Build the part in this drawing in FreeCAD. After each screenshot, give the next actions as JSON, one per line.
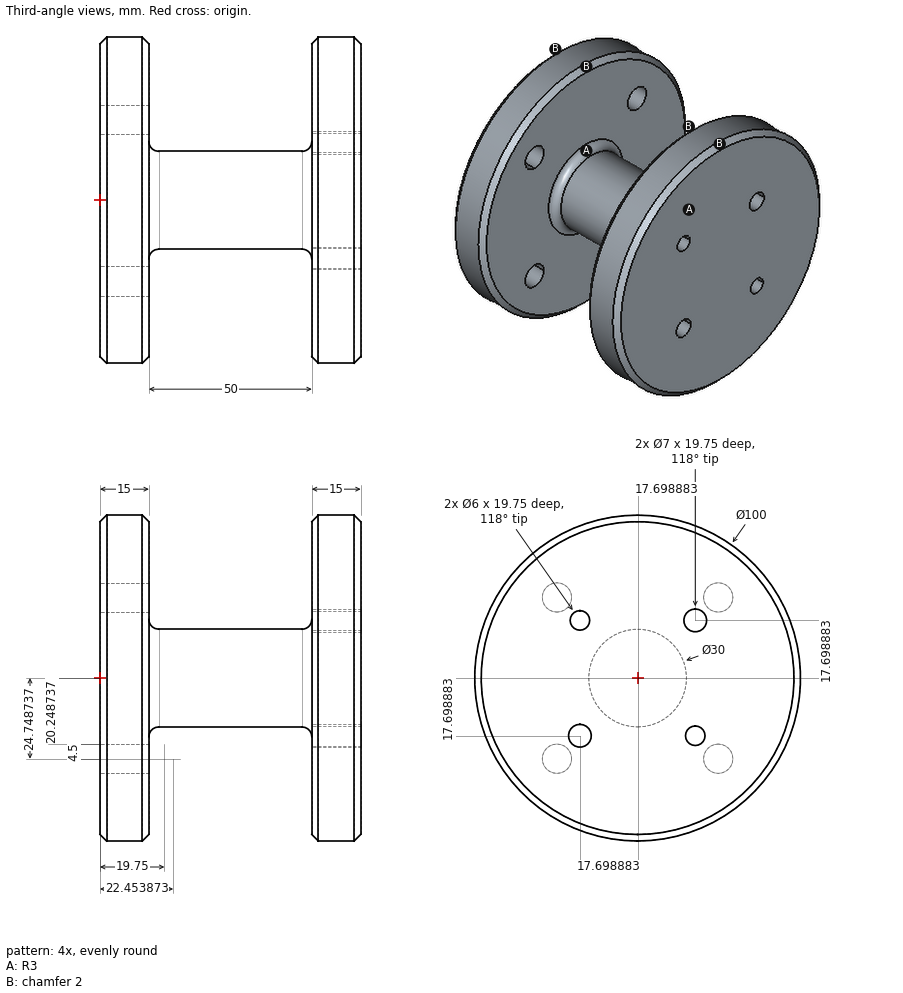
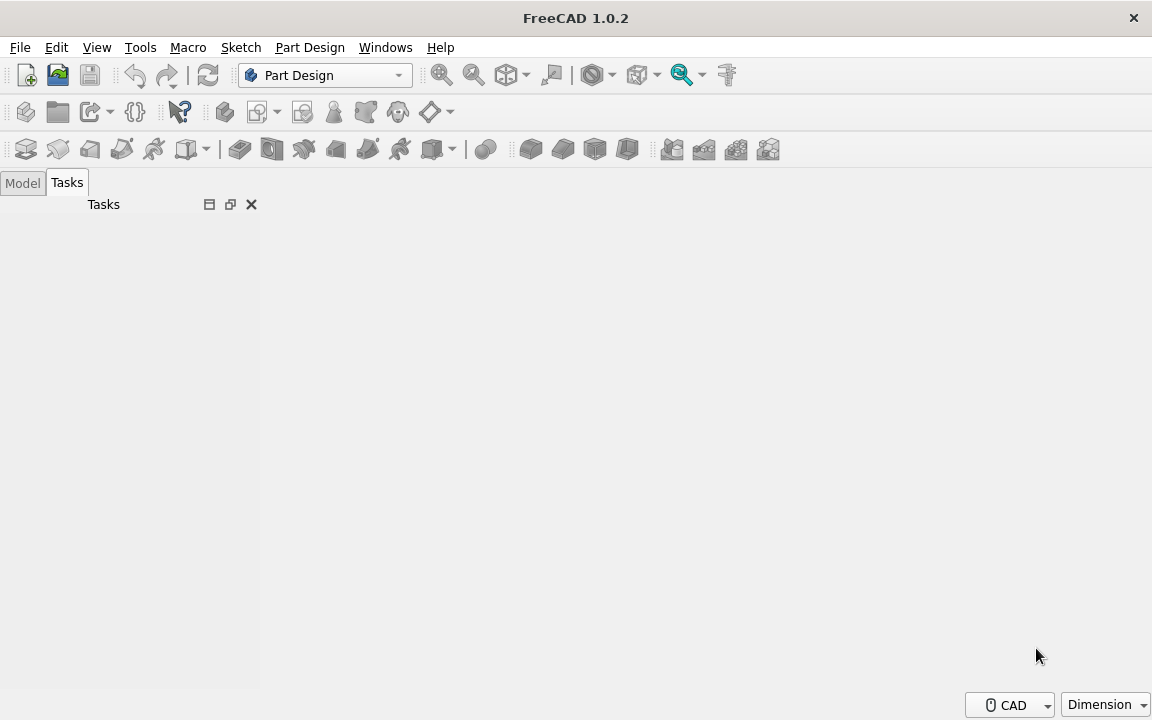
{"action": "left_click", "coordinate": [26, 76]}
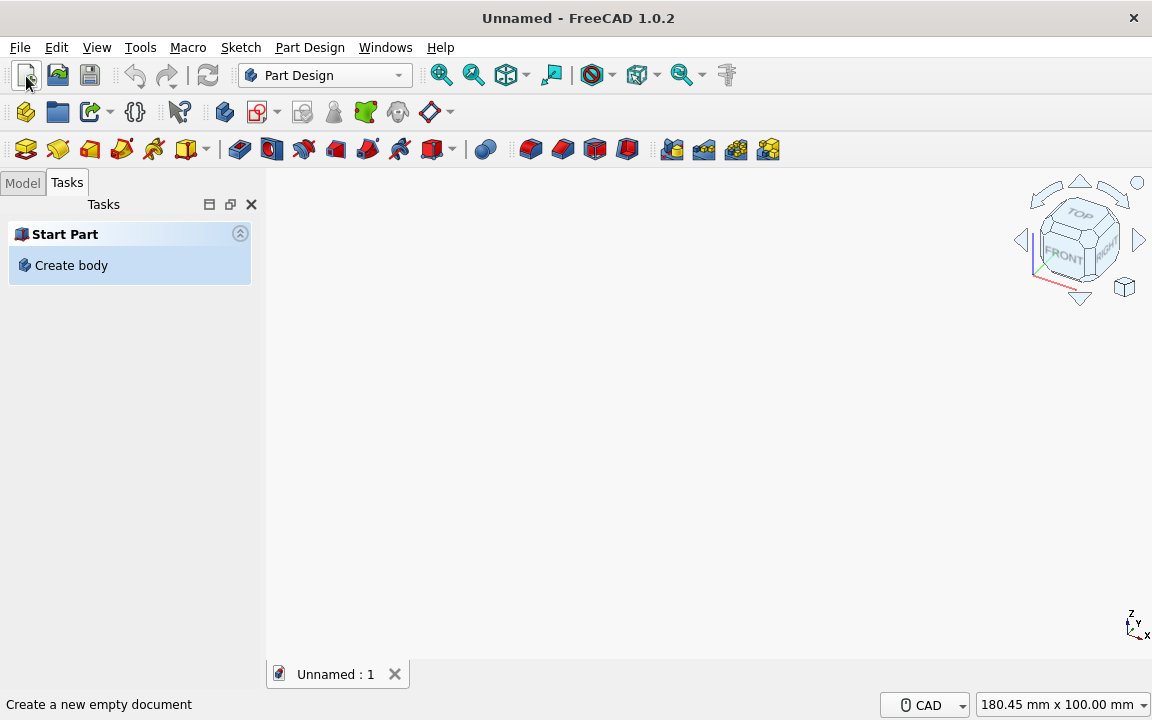
{"action": "left_click", "coordinate": [258, 112]}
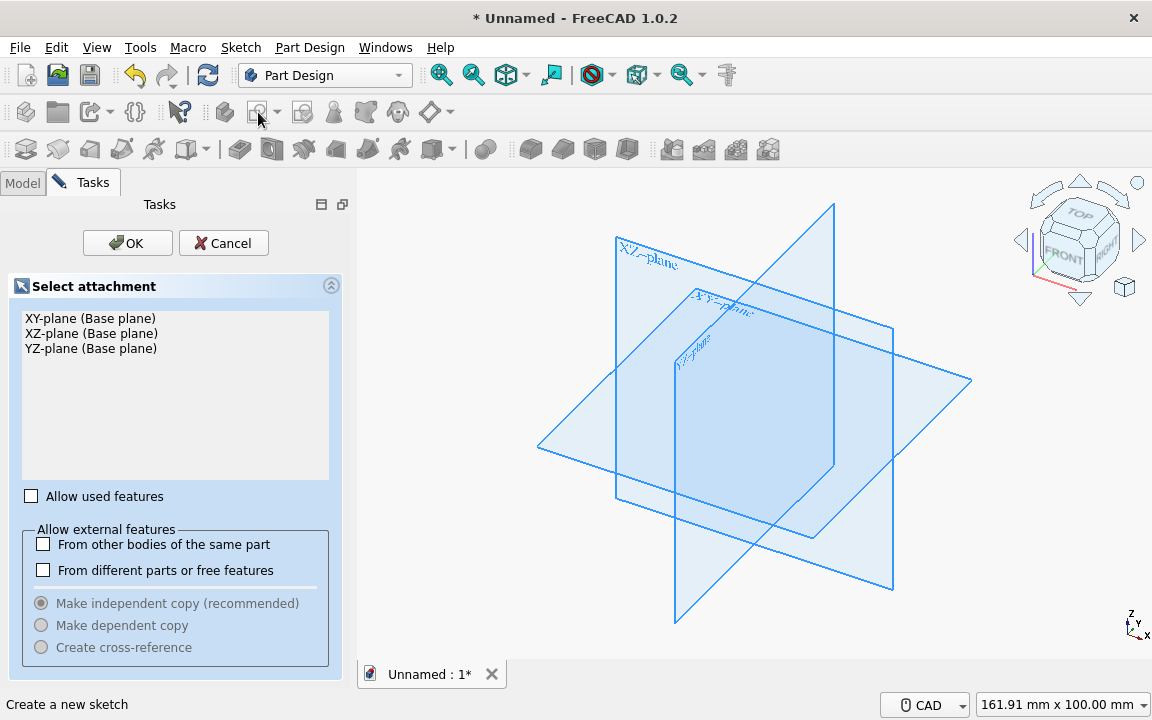
{"action": "left_click", "coordinate": [82, 348]}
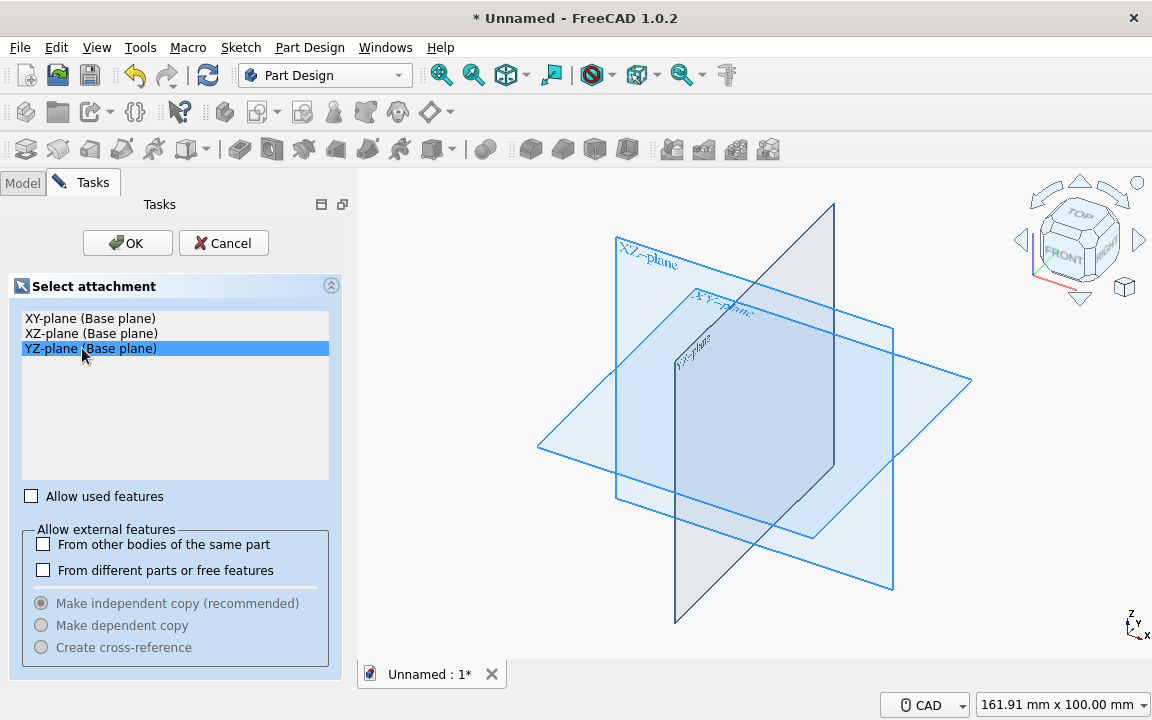
{"action": "left_click", "coordinate": [128, 243]}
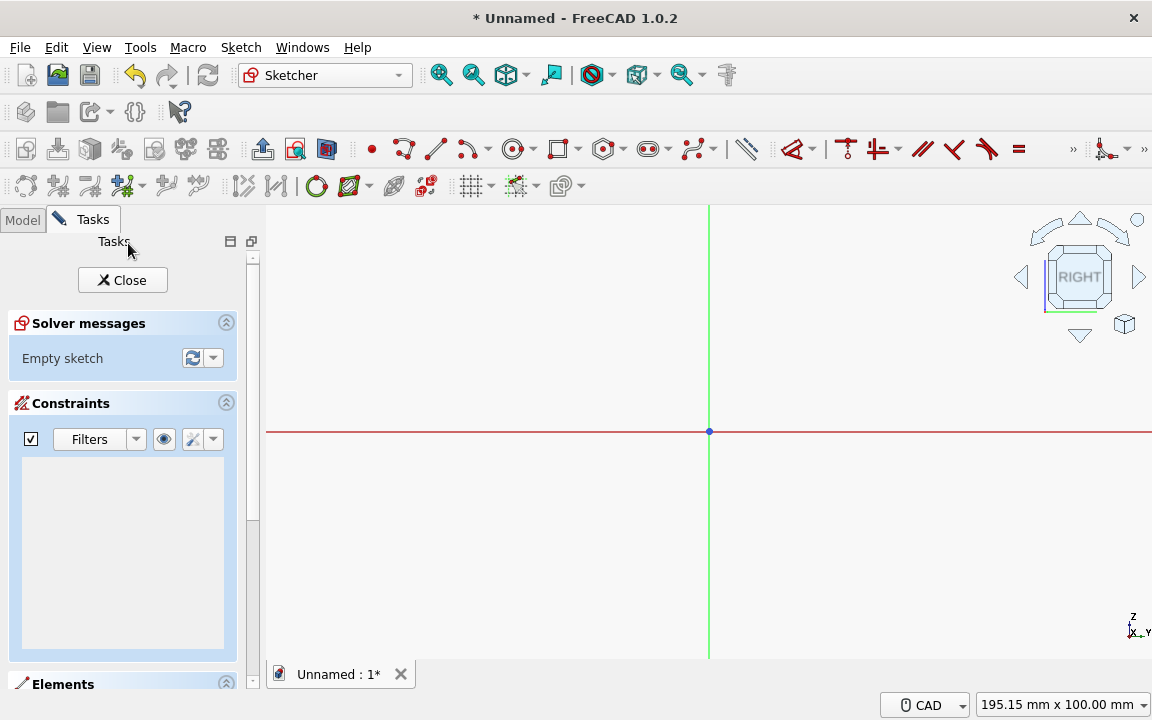
{"action": "scroll", "coordinate": [501, 432], "scroll_direction": "down", "scroll_amount": 2}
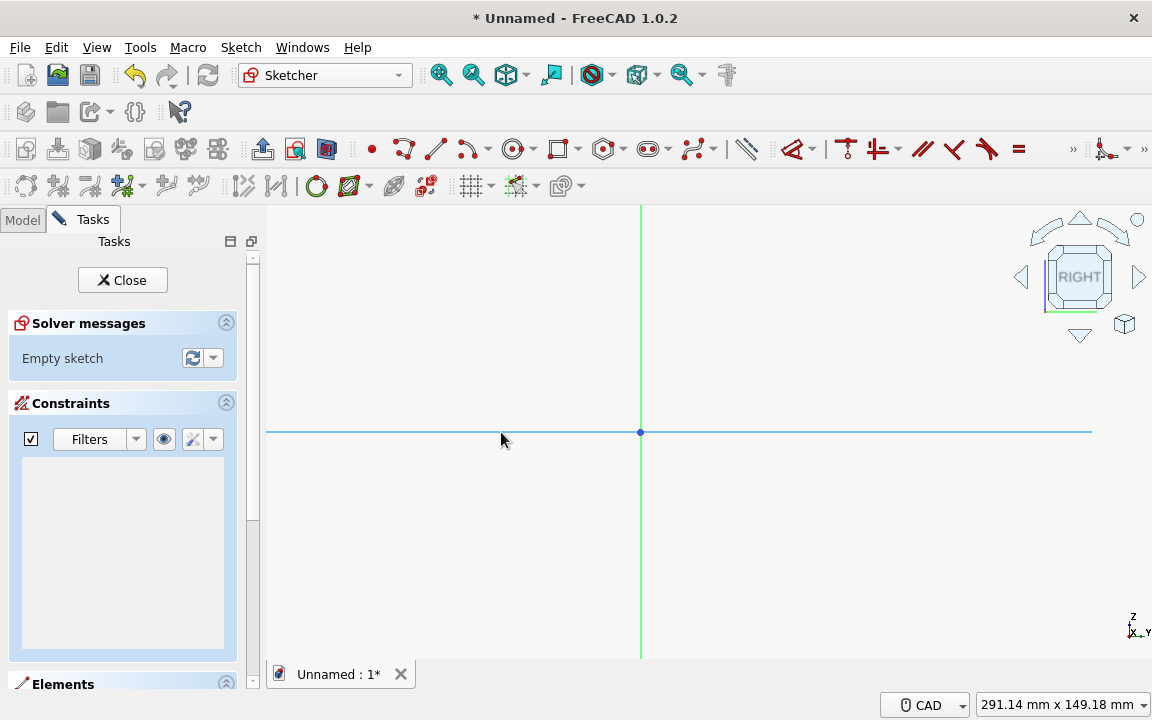
{"action": "left_click", "coordinate": [514, 150]}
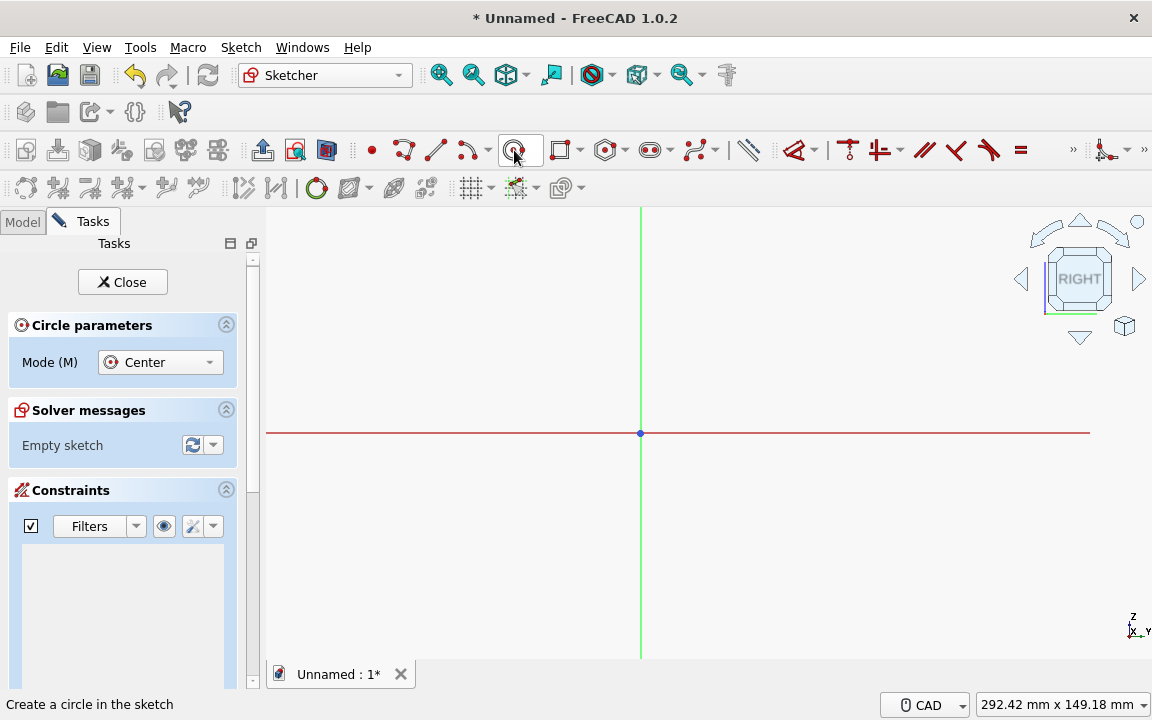
{"action": "left_click", "coordinate": [641, 433]}
{"action": "left_click", "coordinate": [748, 326]}
{"action": "key", "text": "Escape"}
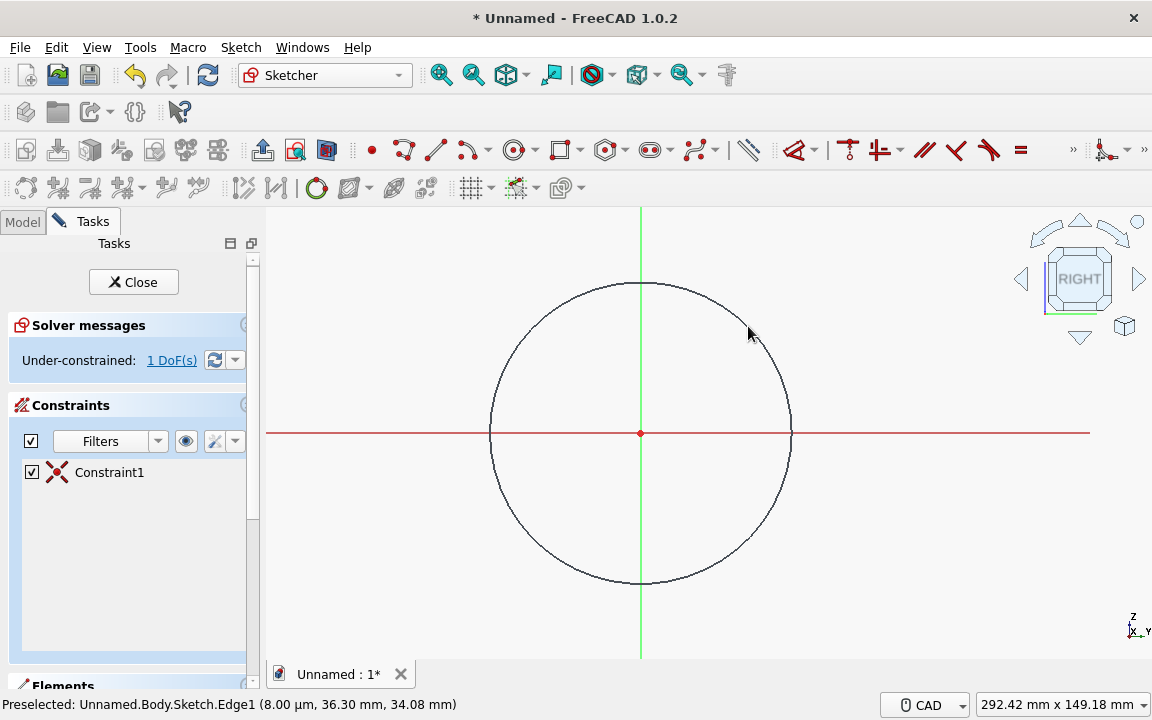
{"action": "left_click", "coordinate": [794, 150]}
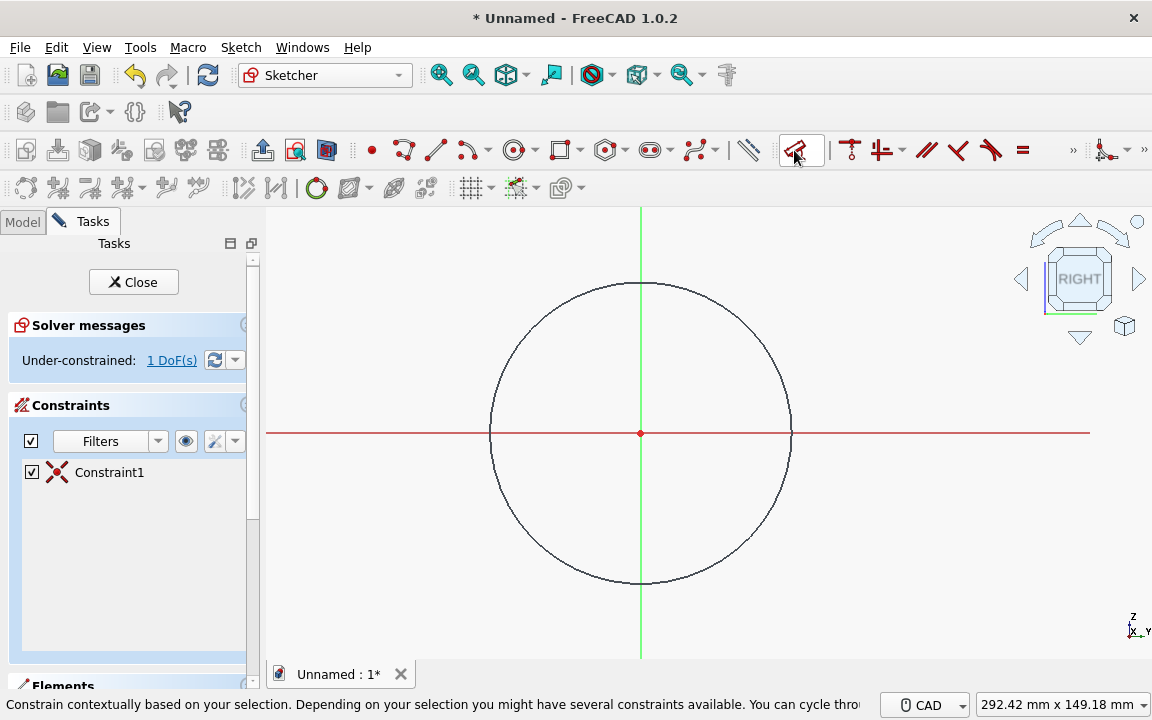
{"action": "left_click", "coordinate": [747, 326]}
{"action": "left_click", "coordinate": [770, 303]}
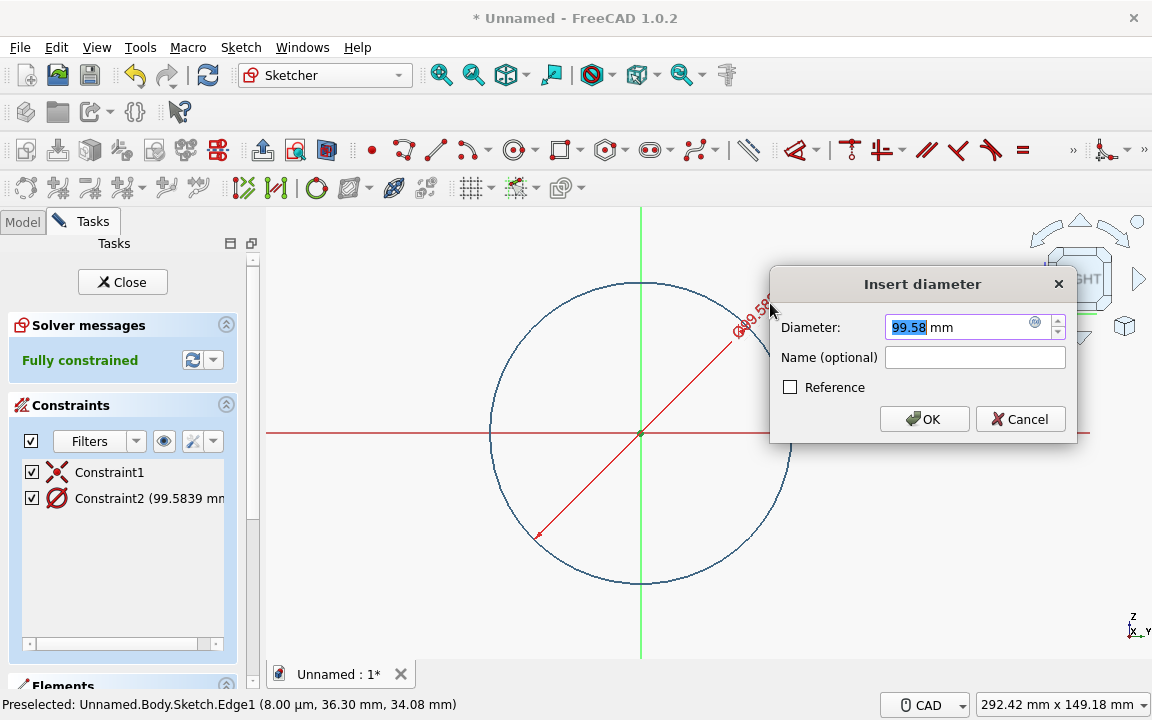
{"action": "type", "text": "100"}
{"action": "key", "text": "Return"}
{"action": "key", "text": "Escape"}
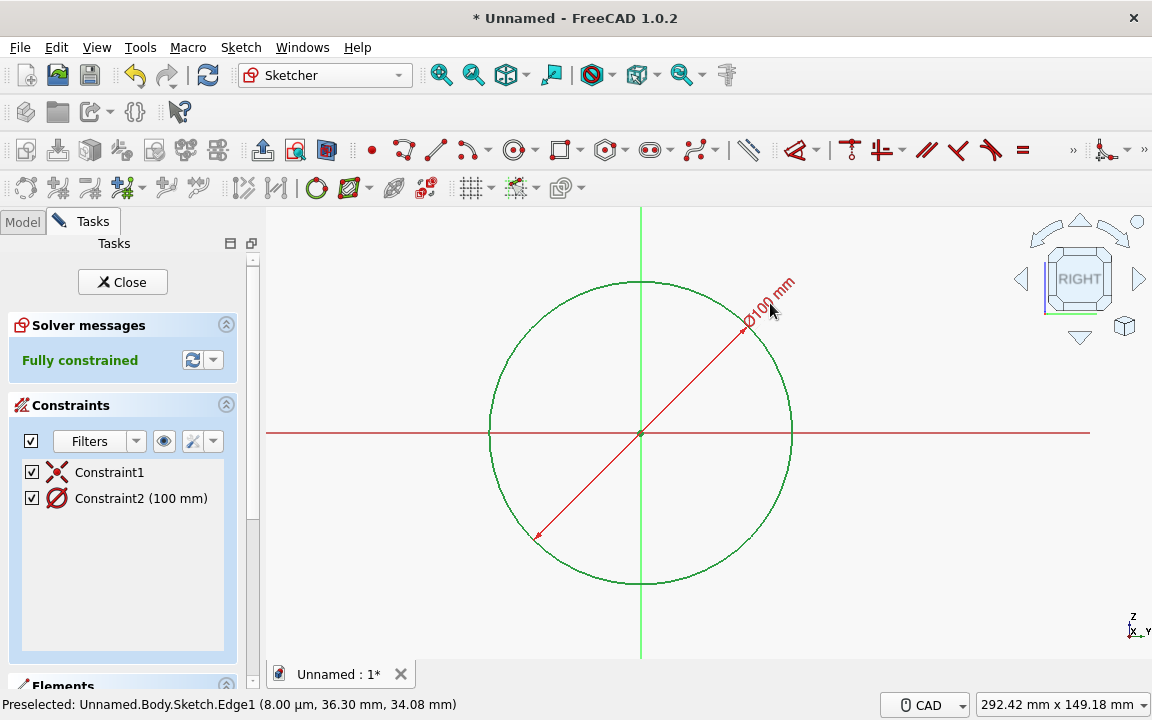
{"action": "left_click", "coordinate": [123, 282]}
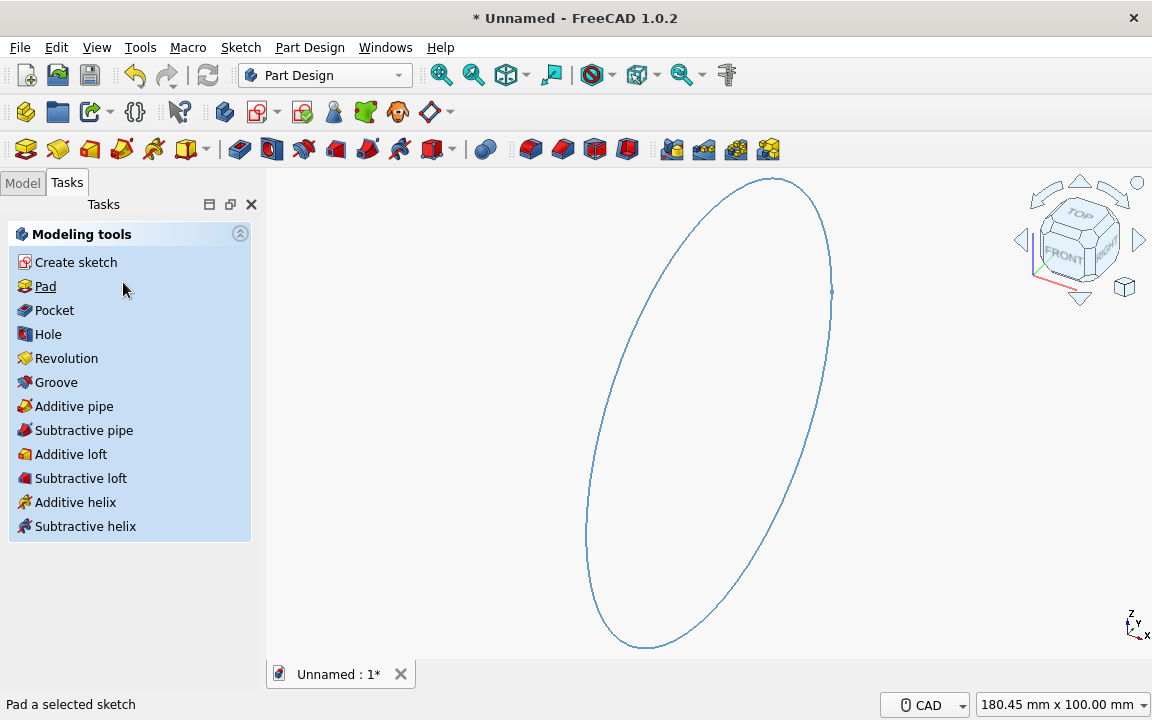
{"action": "left_click", "coordinate": [26, 150]}